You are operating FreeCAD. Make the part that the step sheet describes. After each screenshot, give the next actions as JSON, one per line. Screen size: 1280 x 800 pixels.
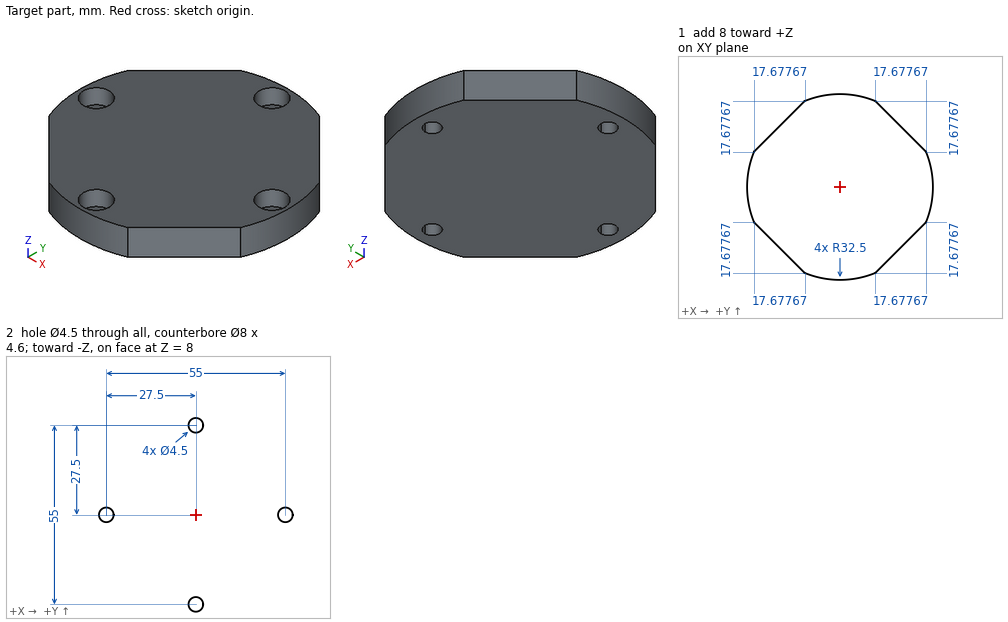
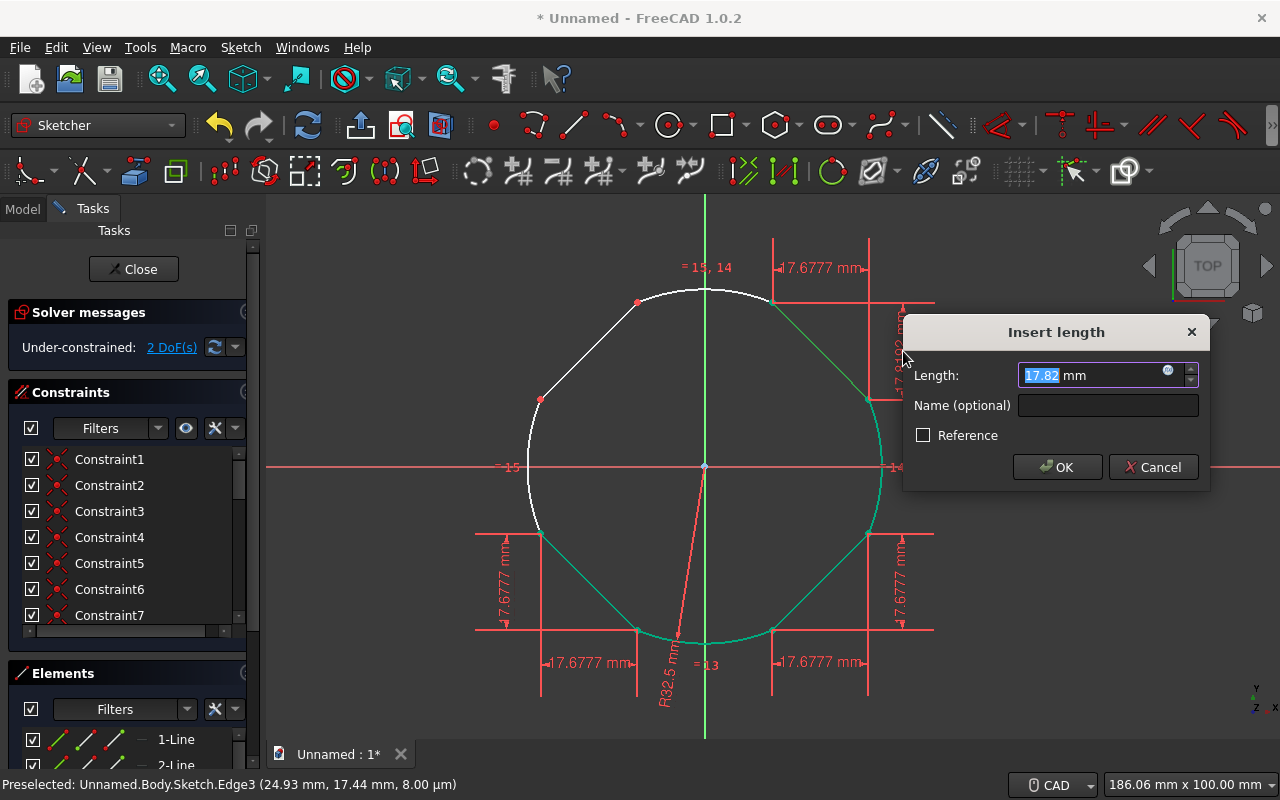
{"action": "type", "text": "17.67767"}
{"action": "key", "text": "Return"}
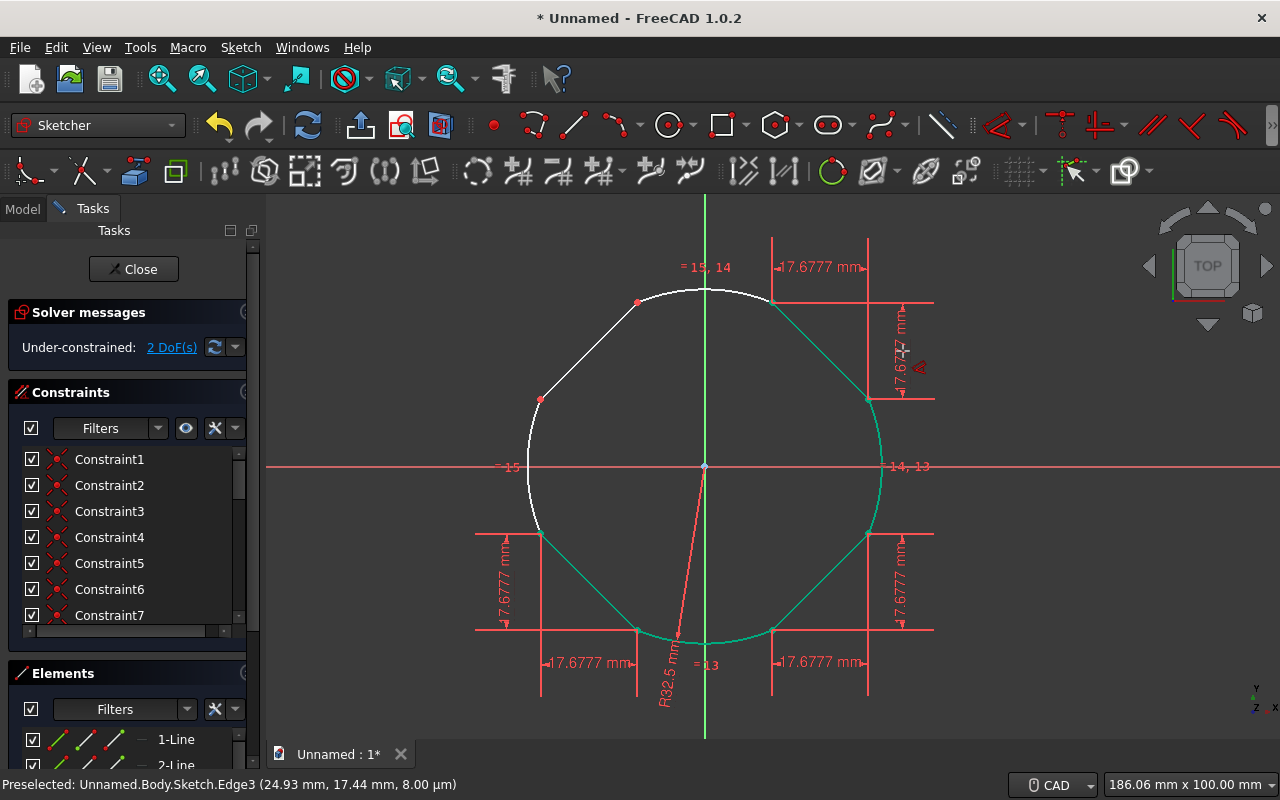
{"action": "left_click", "coordinate": [608, 332]}
{"action": "left_click", "coordinate": [589, 269]}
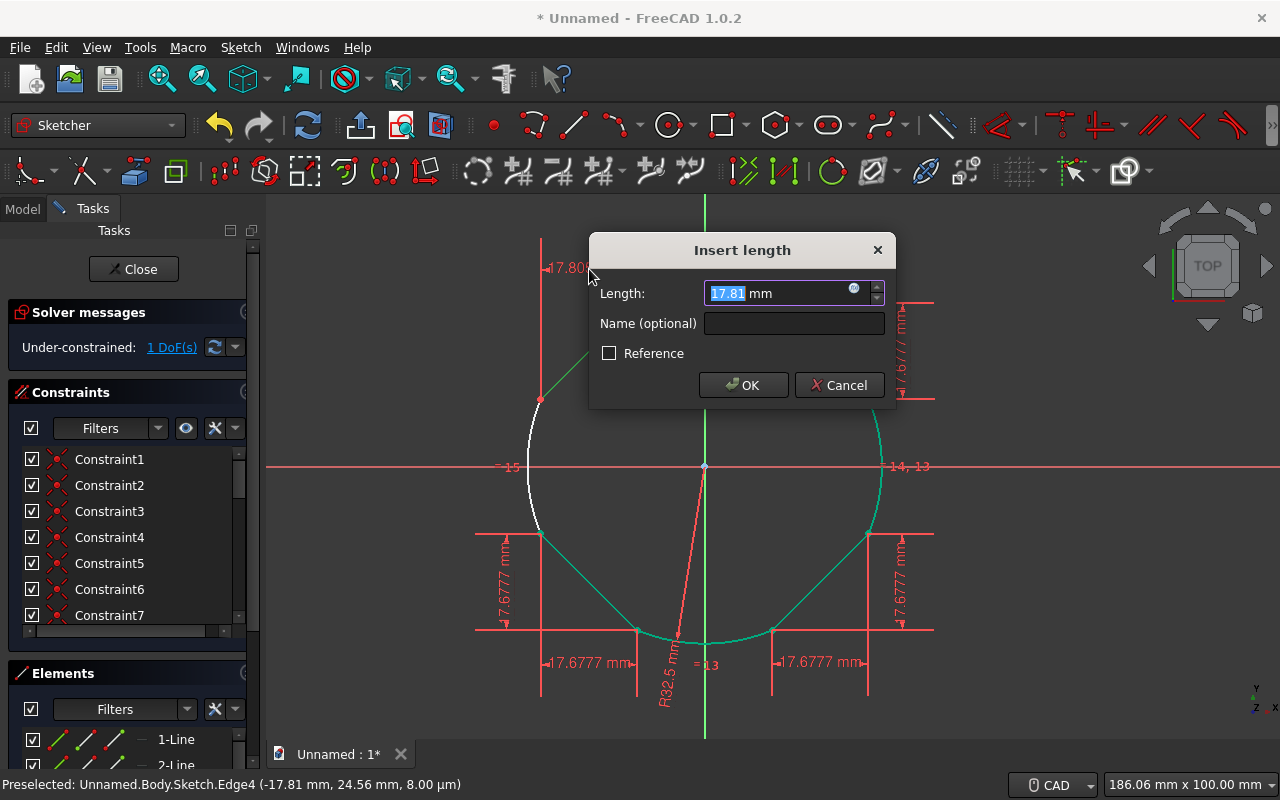
{"action": "type", "text": "17.67767"}
{"action": "key", "text": "Return"}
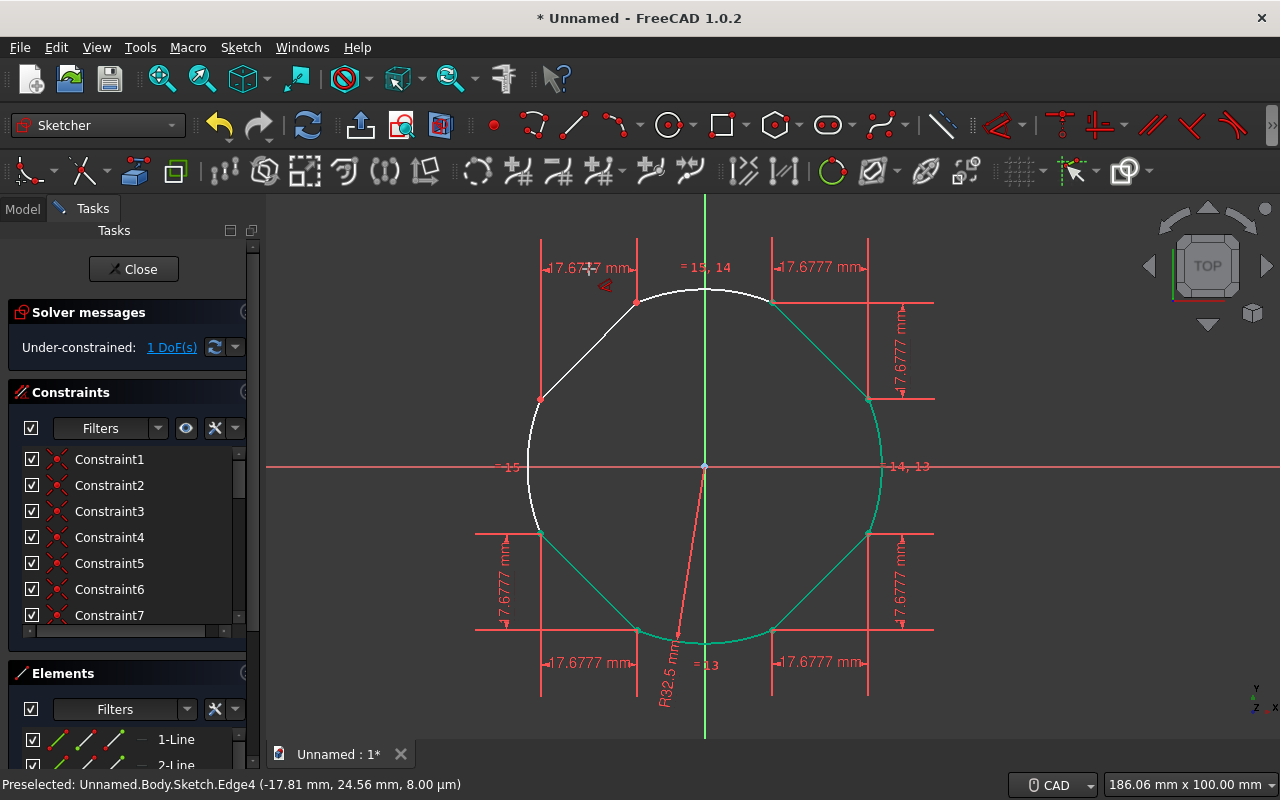
{"action": "left_click", "coordinate": [608, 332]}
{"action": "left_click", "coordinate": [507, 351]}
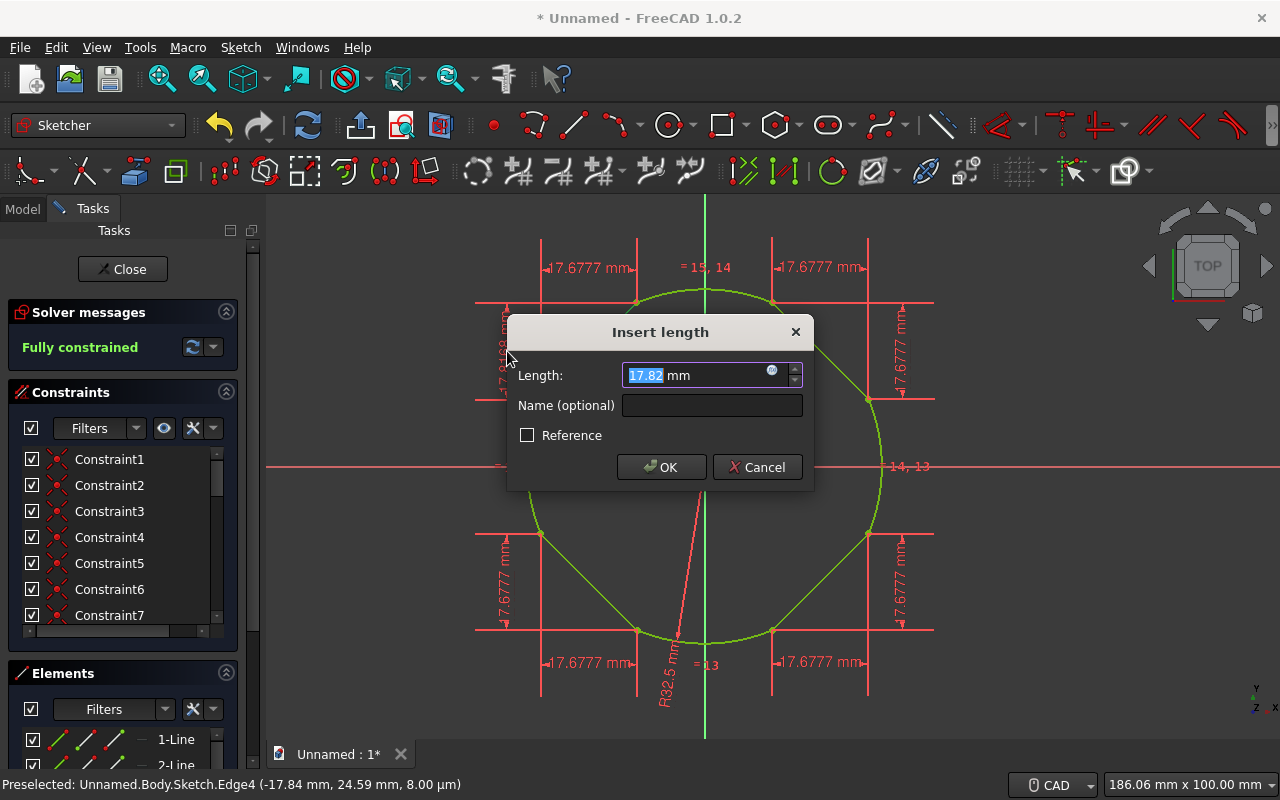
{"action": "type", "text": "17.67767"}
{"action": "key", "text": "Return"}
{"action": "key", "text": "Escape"}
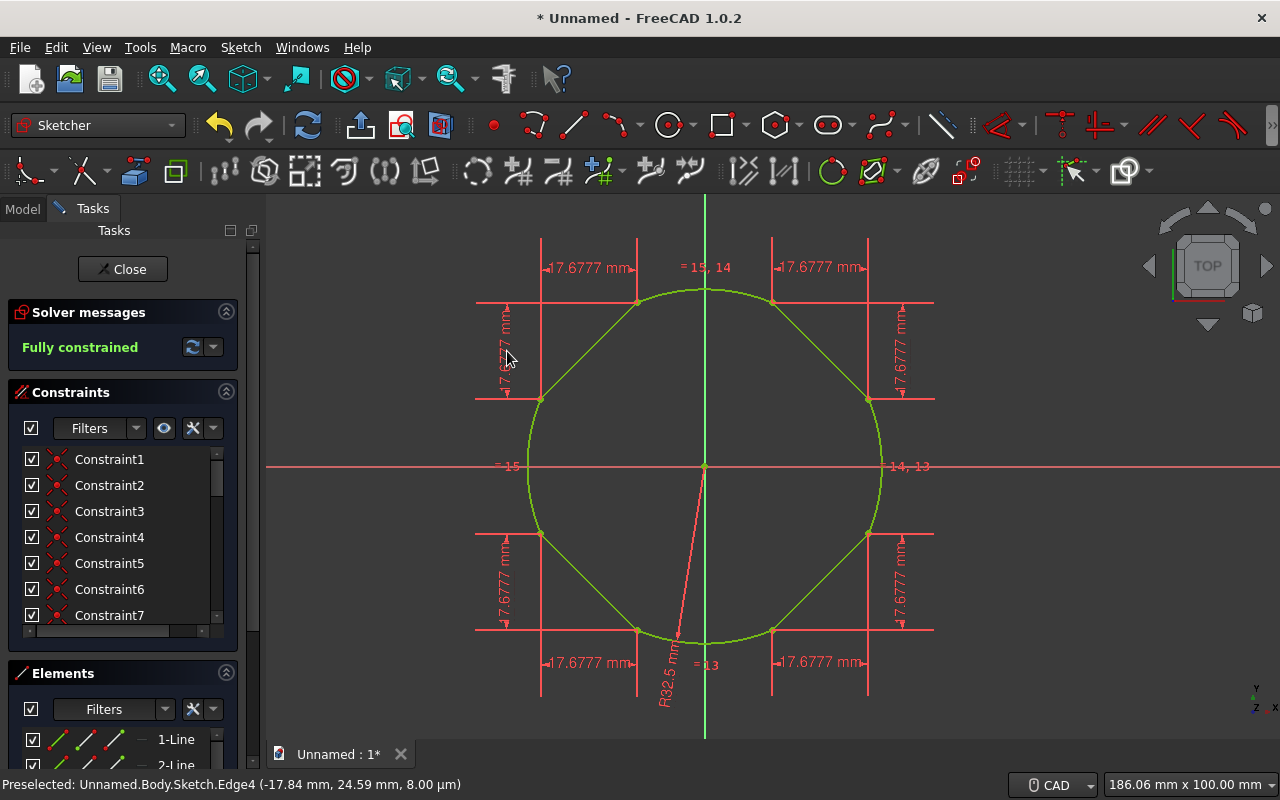
{"action": "left_click", "coordinate": [123, 269]}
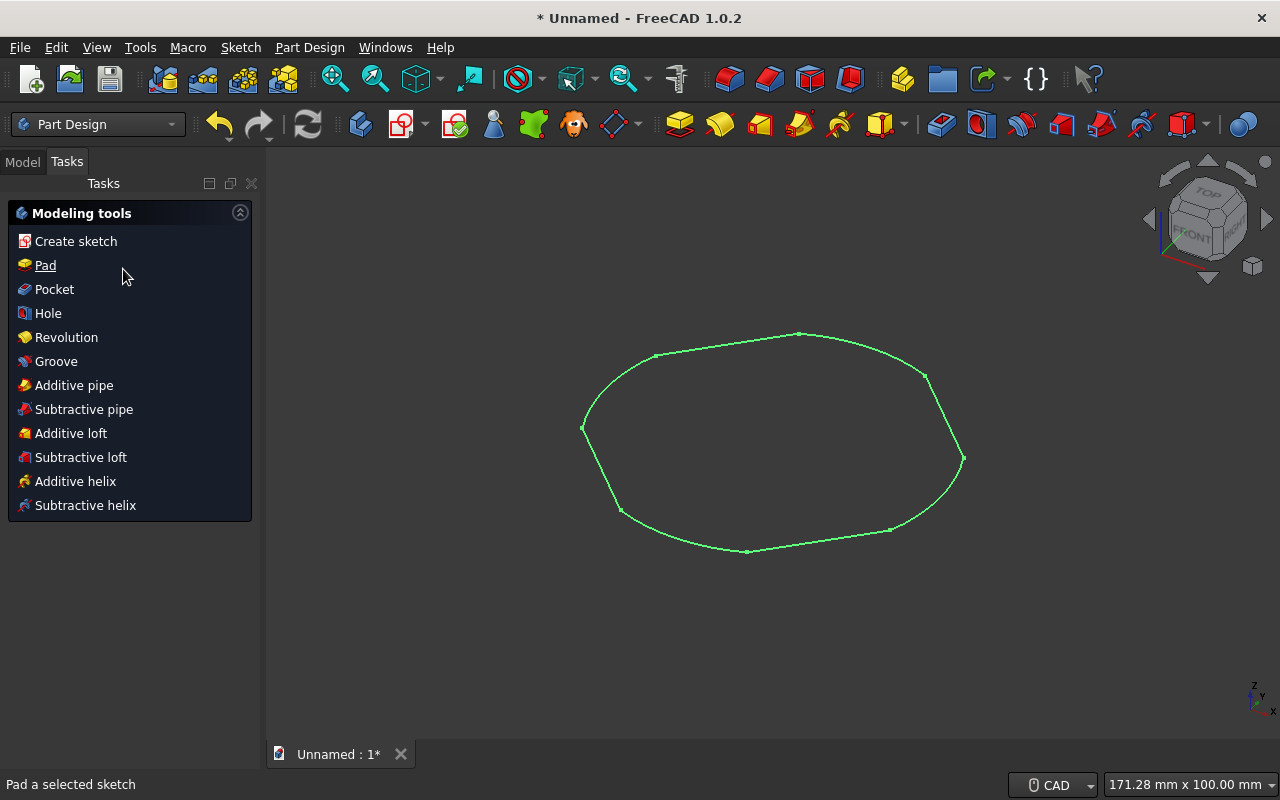
{"action": "left_click", "coordinate": [680, 124]}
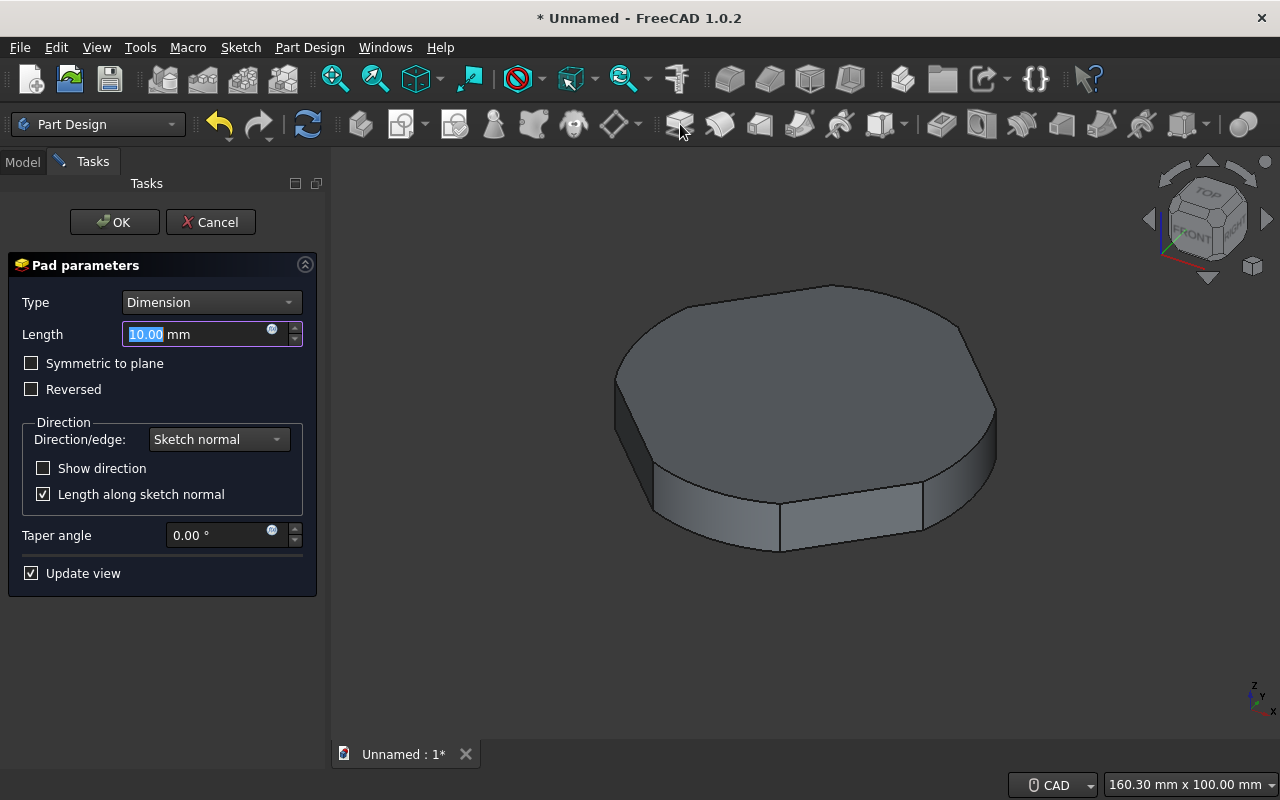
{"action": "type", "text": "8"}
{"action": "key", "text": "Tab"}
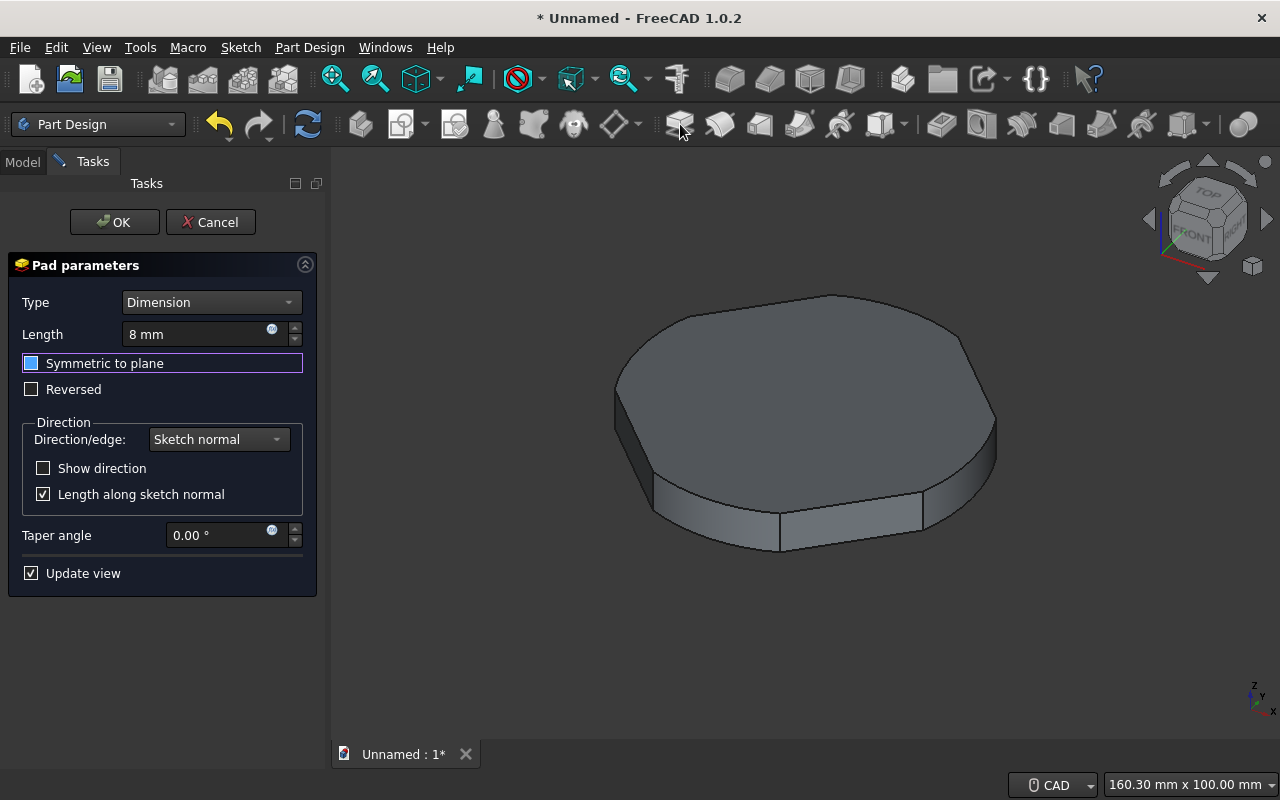
{"action": "left_click", "coordinate": [115, 222]}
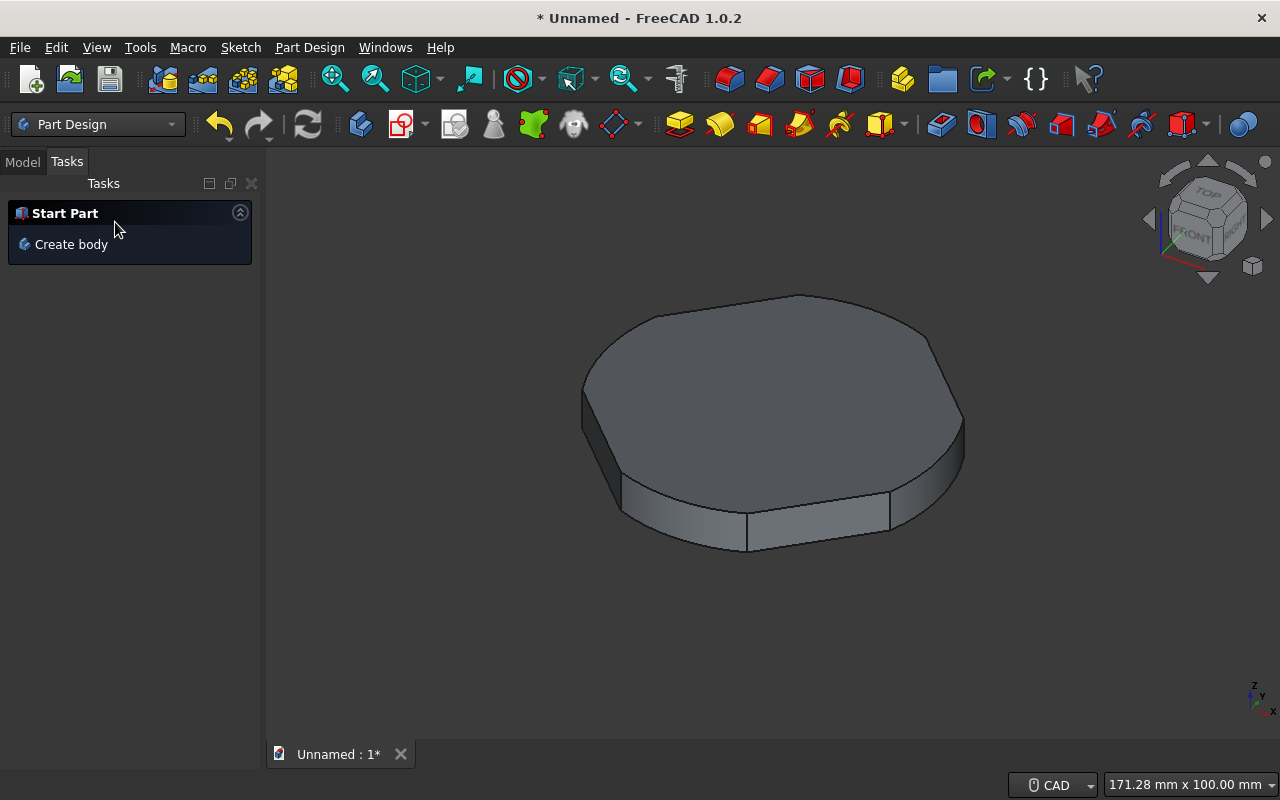
{"action": "left_click", "coordinate": [773, 403]}